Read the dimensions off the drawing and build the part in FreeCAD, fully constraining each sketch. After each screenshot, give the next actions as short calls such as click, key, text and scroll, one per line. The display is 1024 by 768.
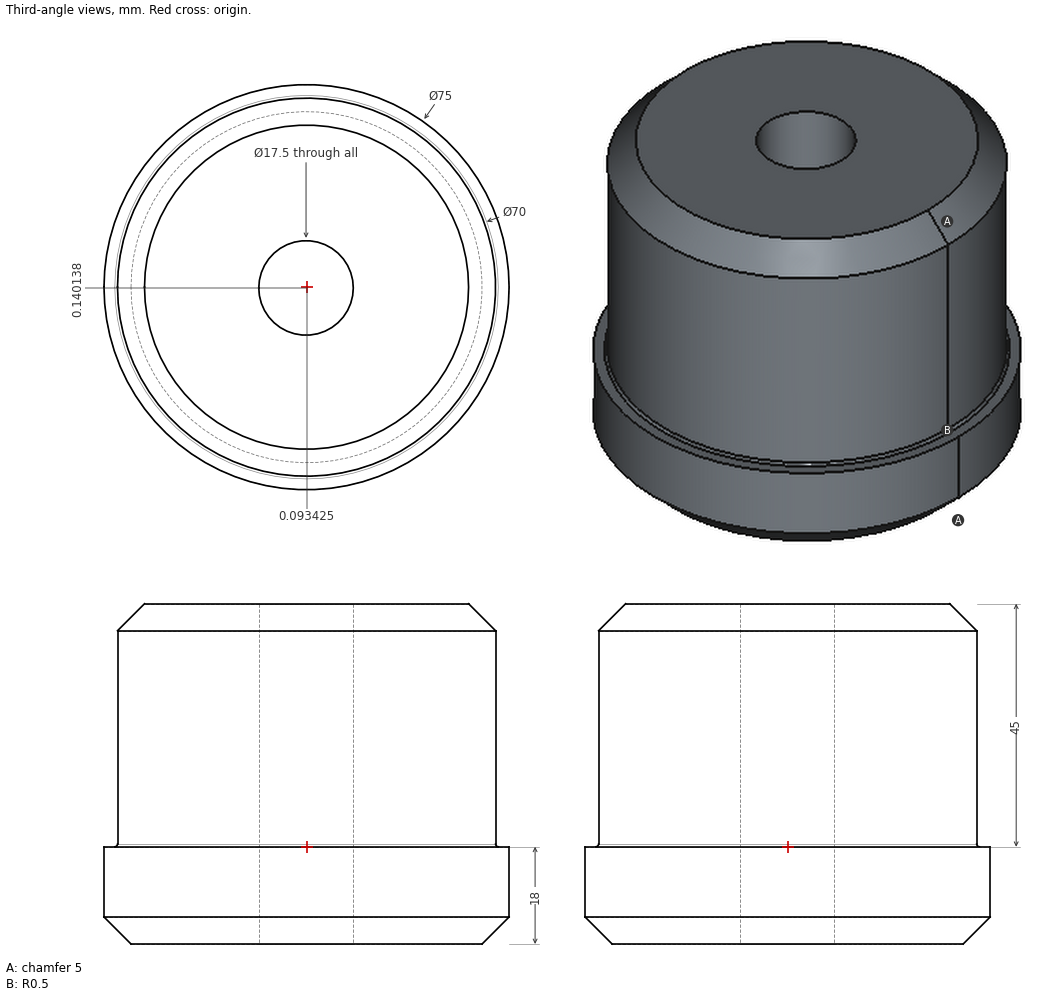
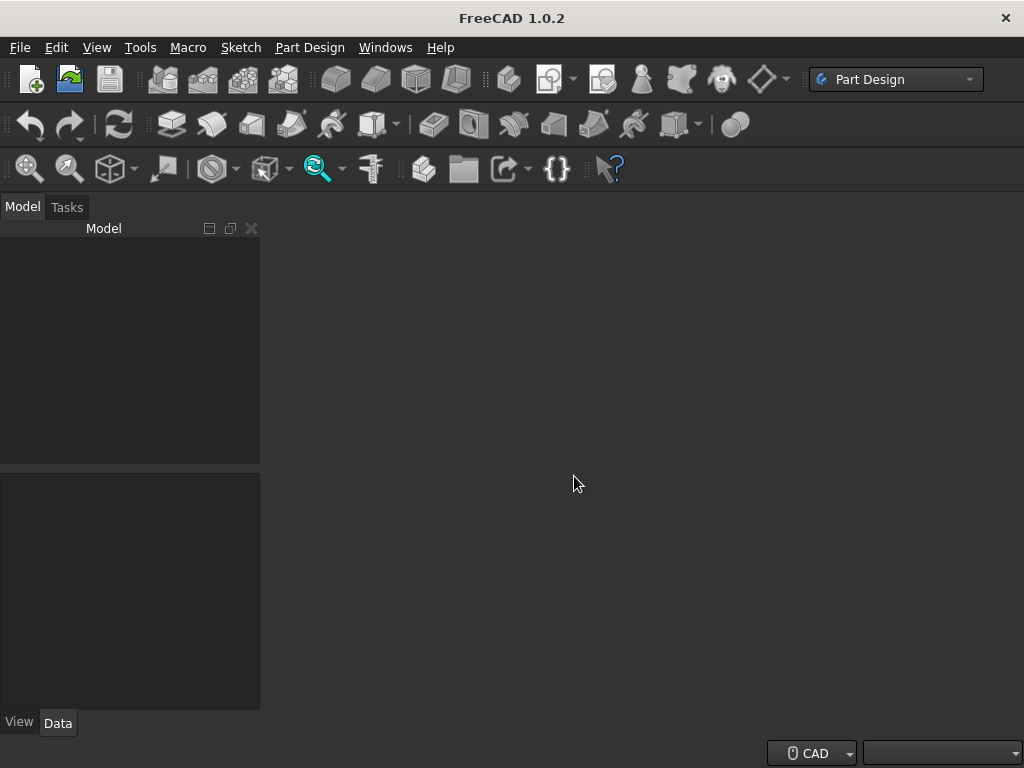
click(30, 80)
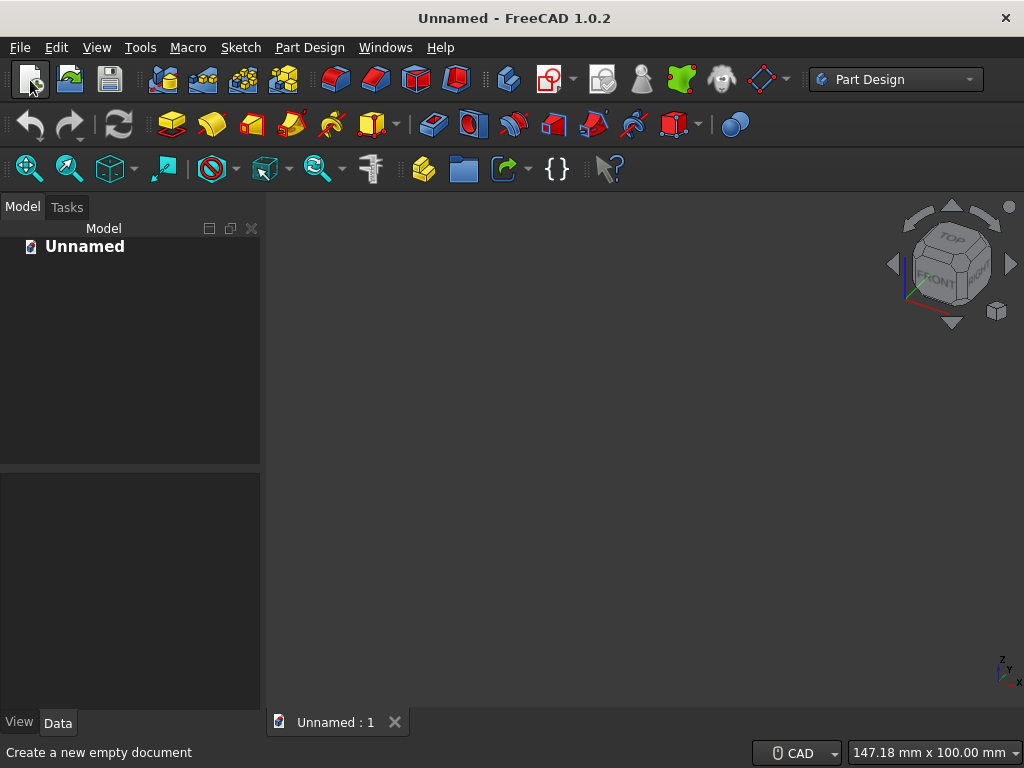
click(550, 80)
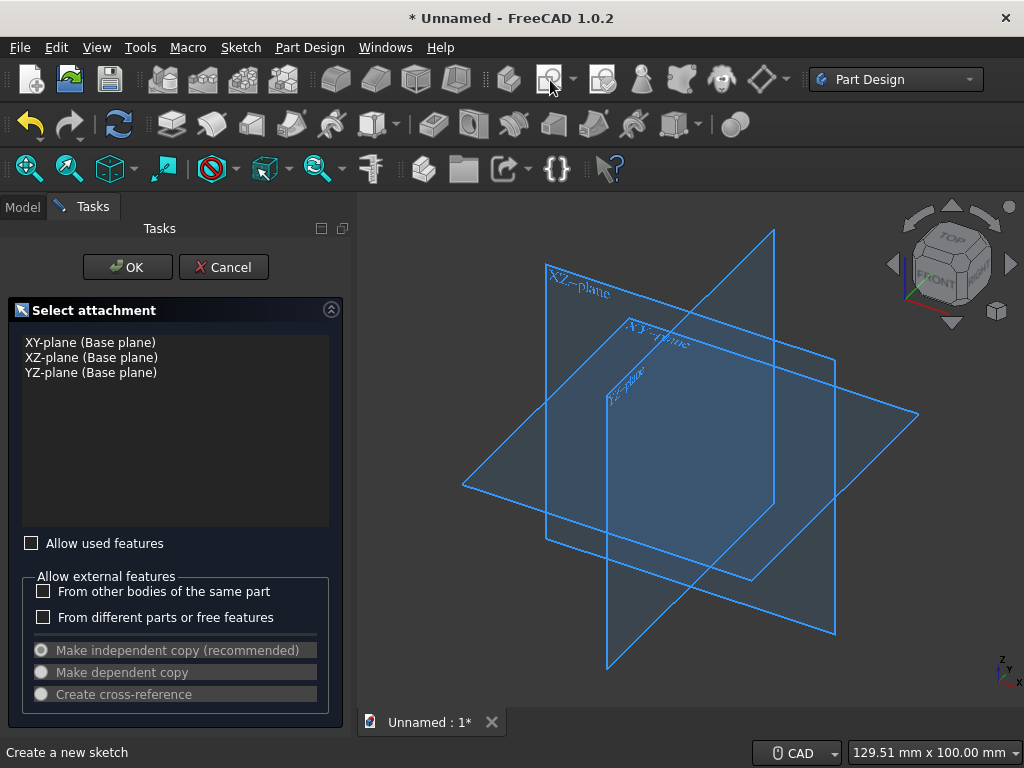
click(82, 342)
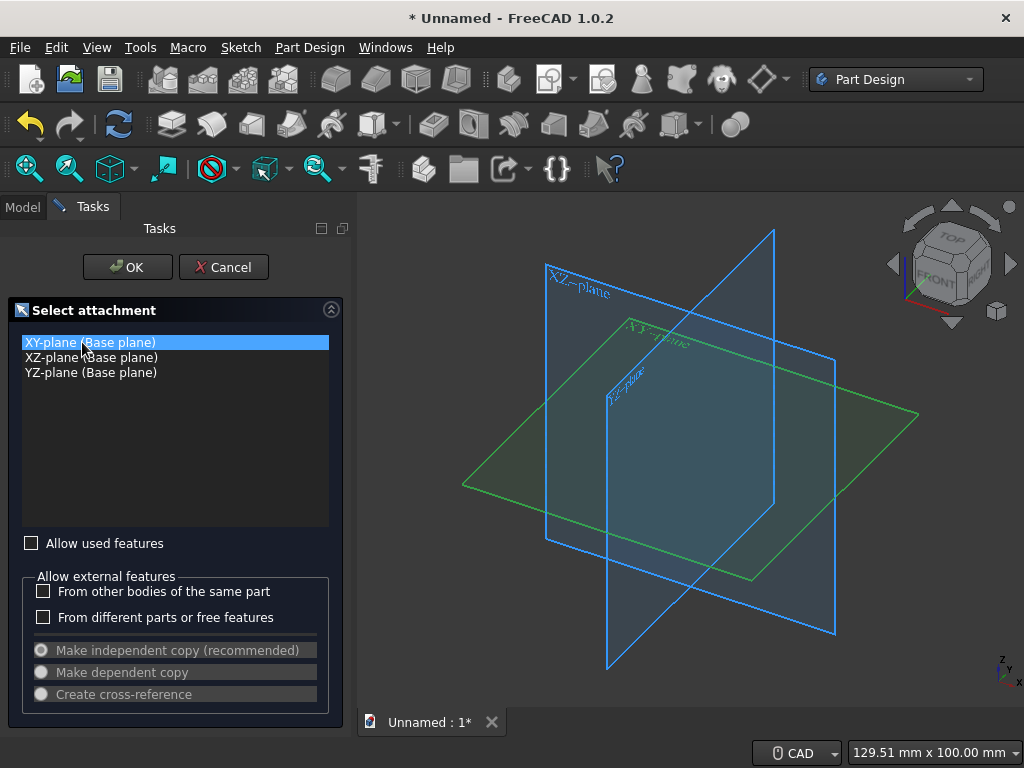
click(128, 267)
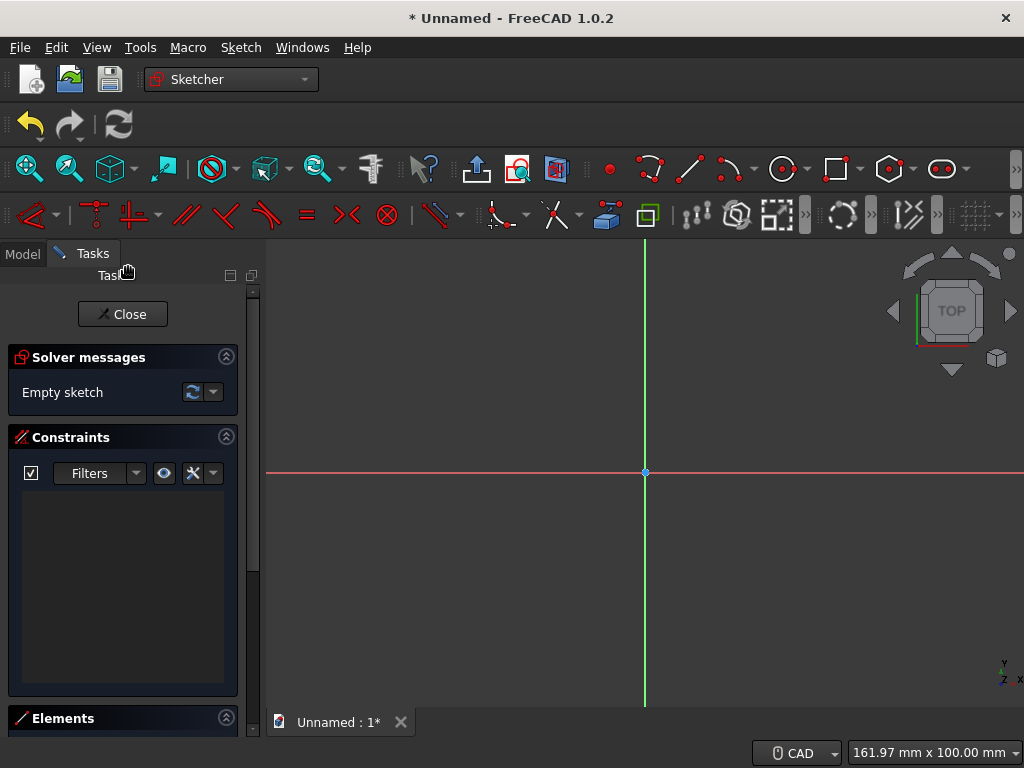
click(784, 170)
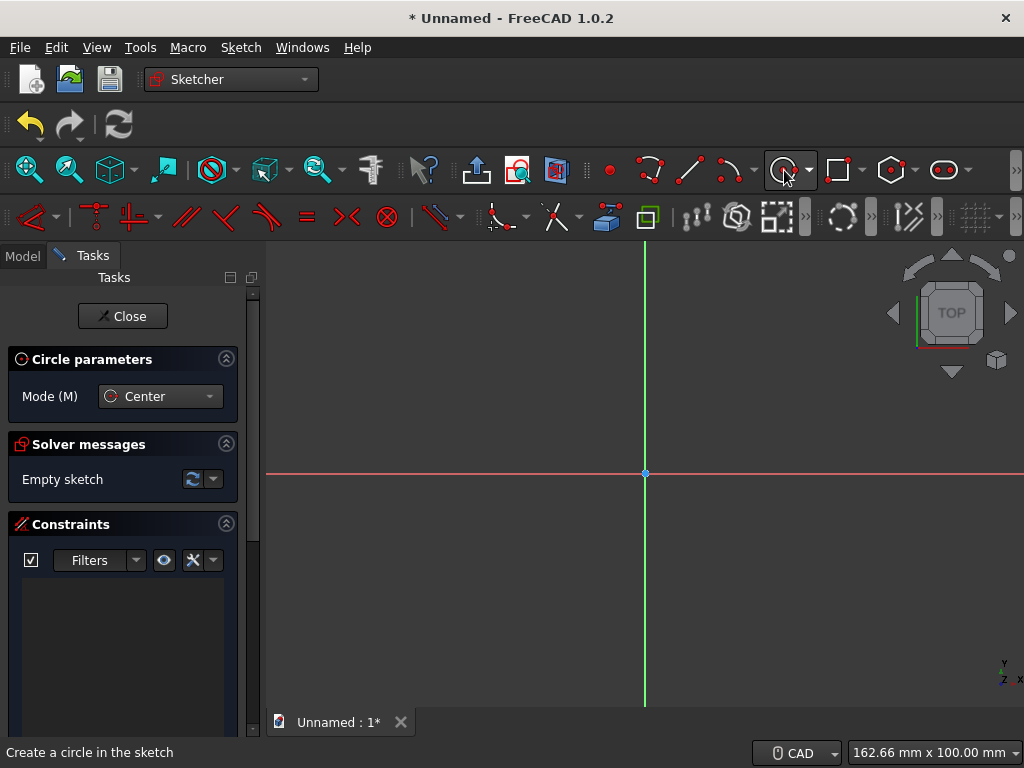
click(645, 474)
click(760, 359)
key(Escape)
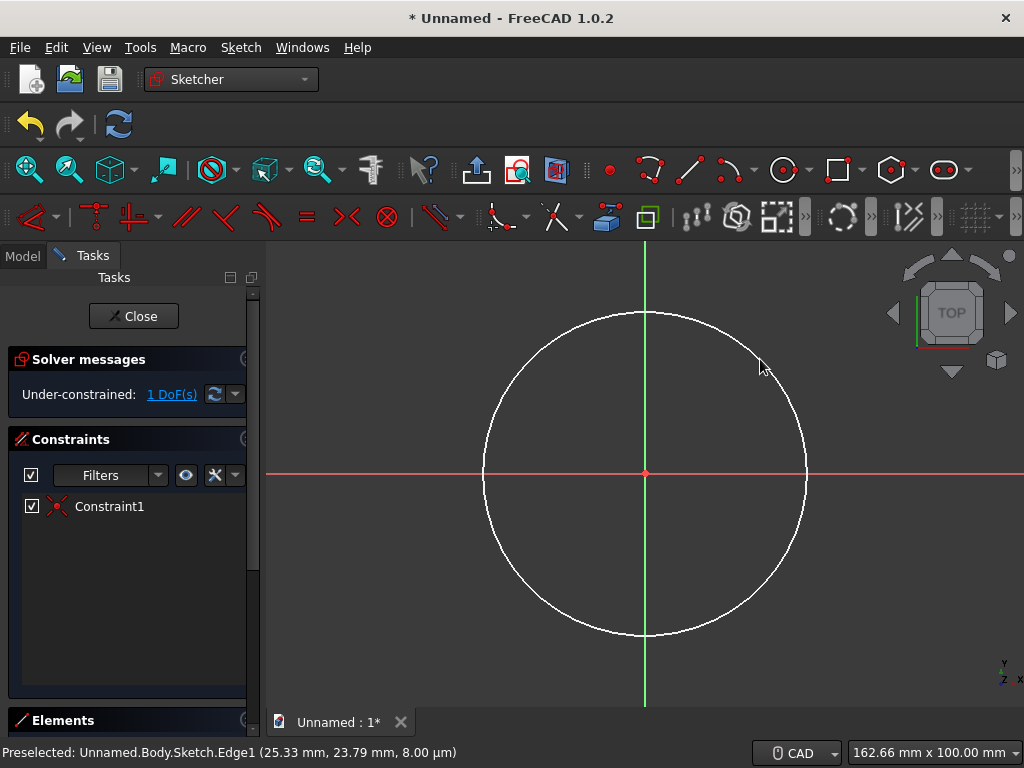
click(759, 359)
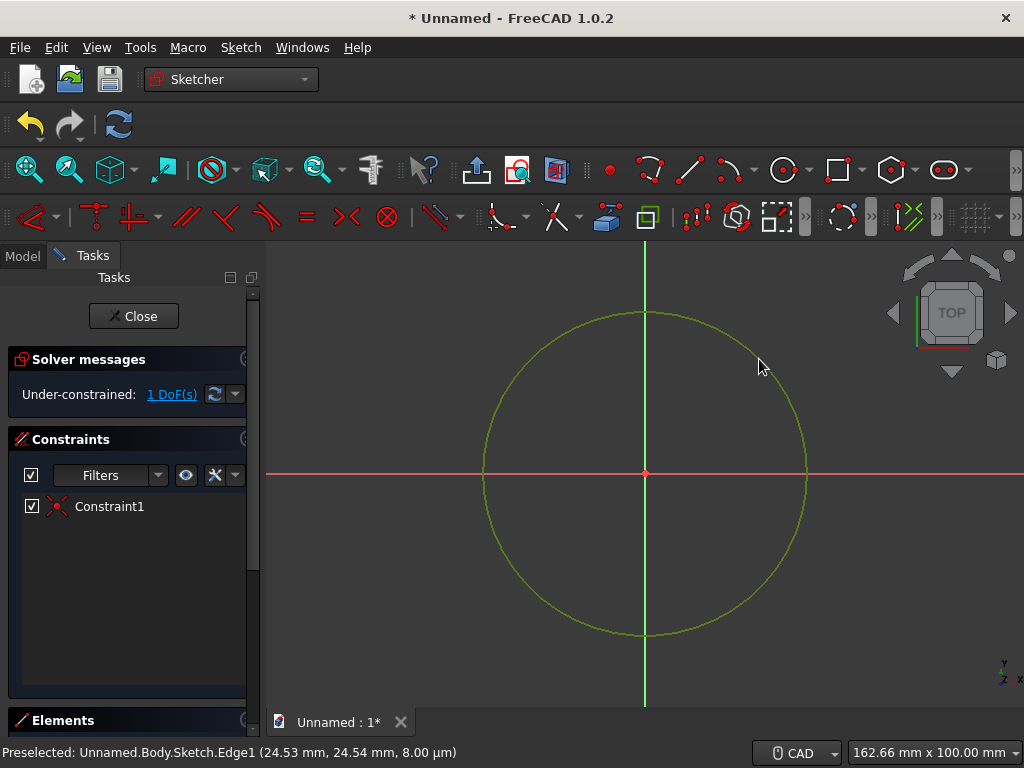
click(58, 218)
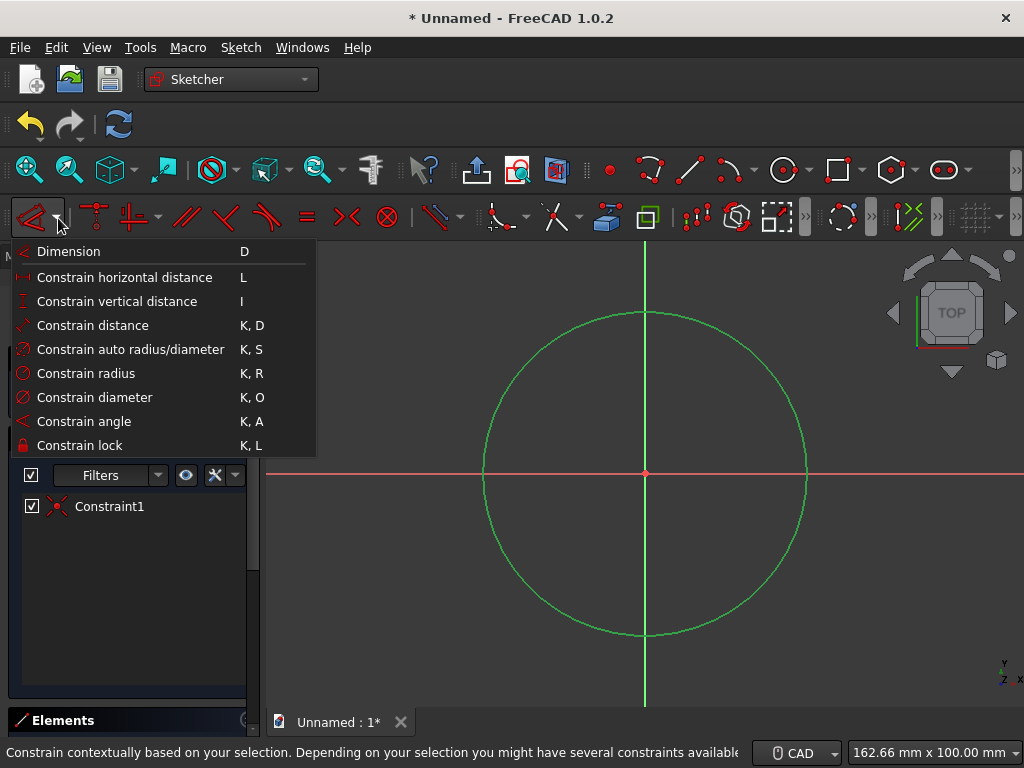
click(164, 397)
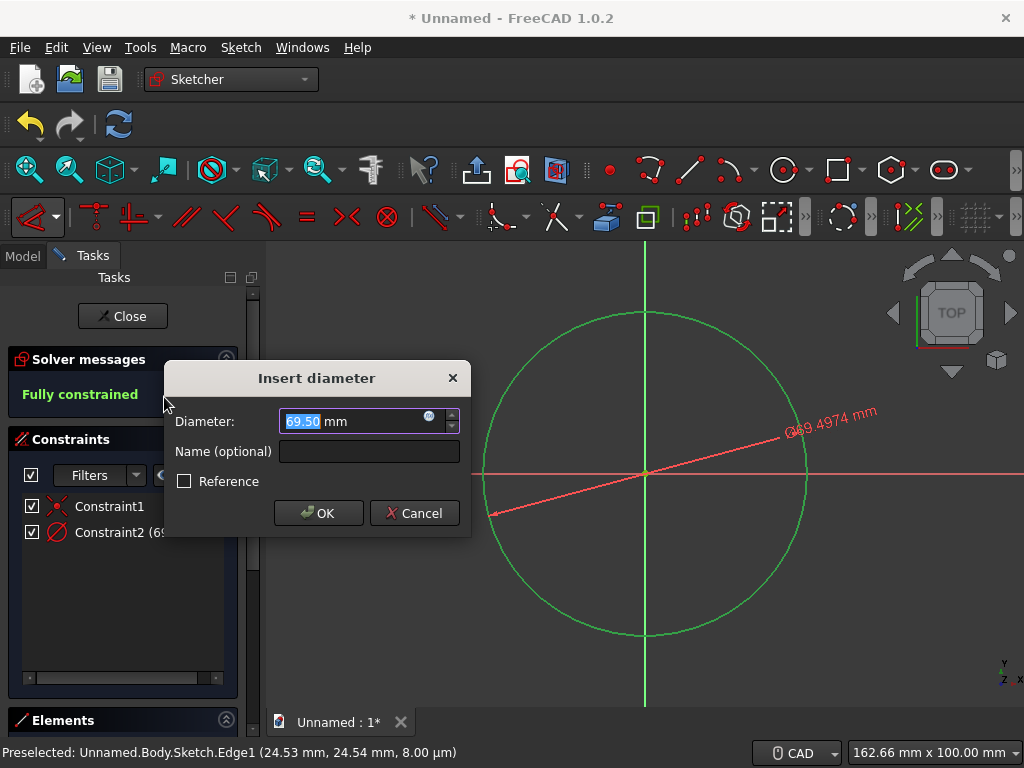
text(70)
key(Return)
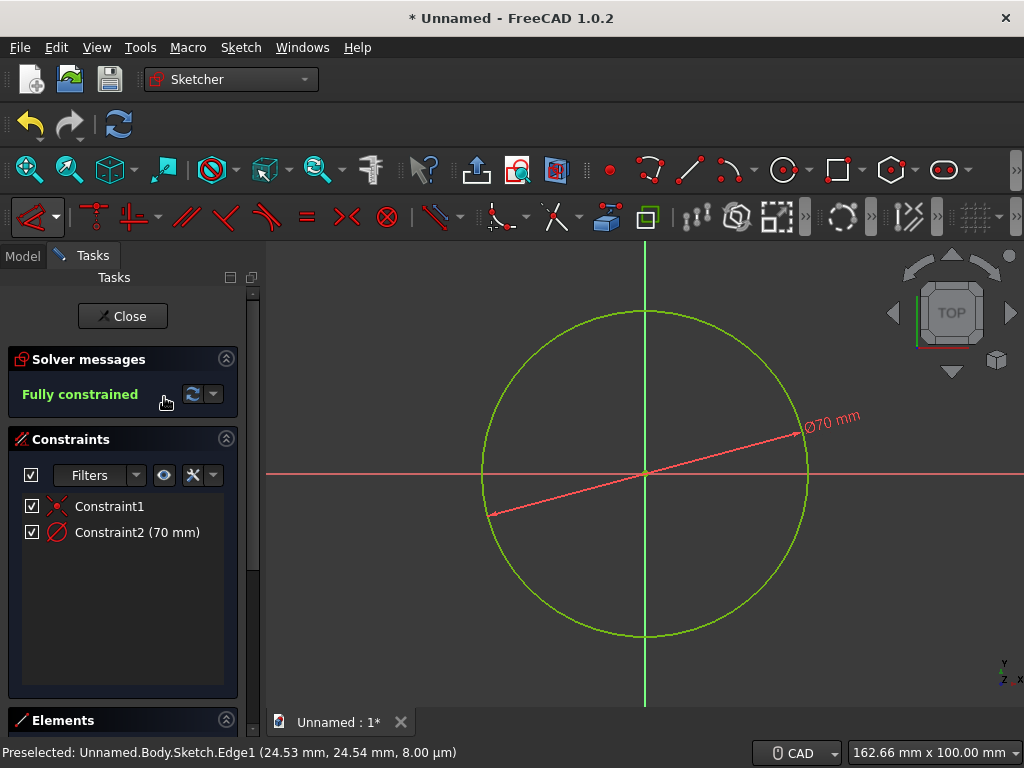
click(123, 316)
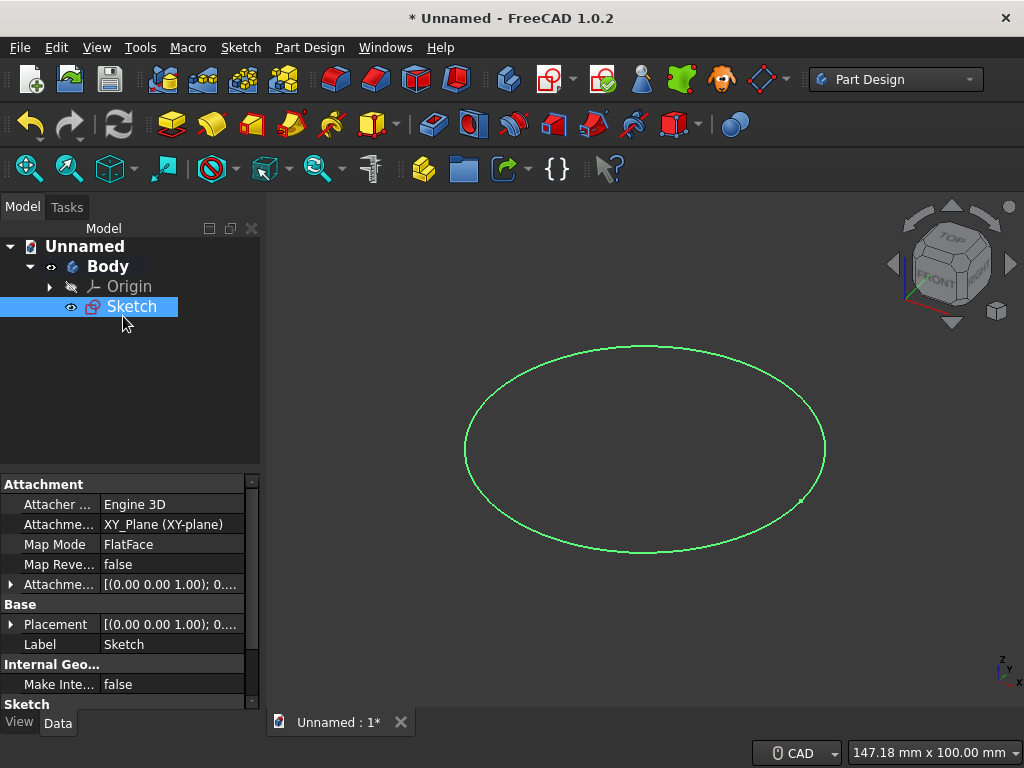
click(172, 124)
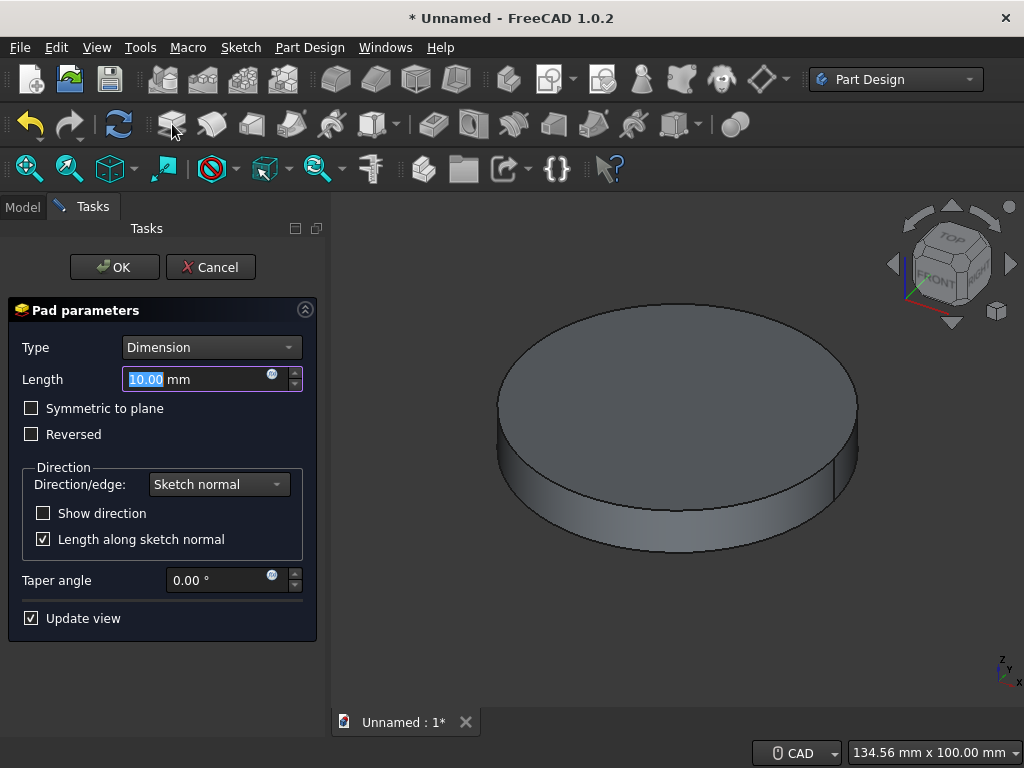
text(45)
key(Tab)